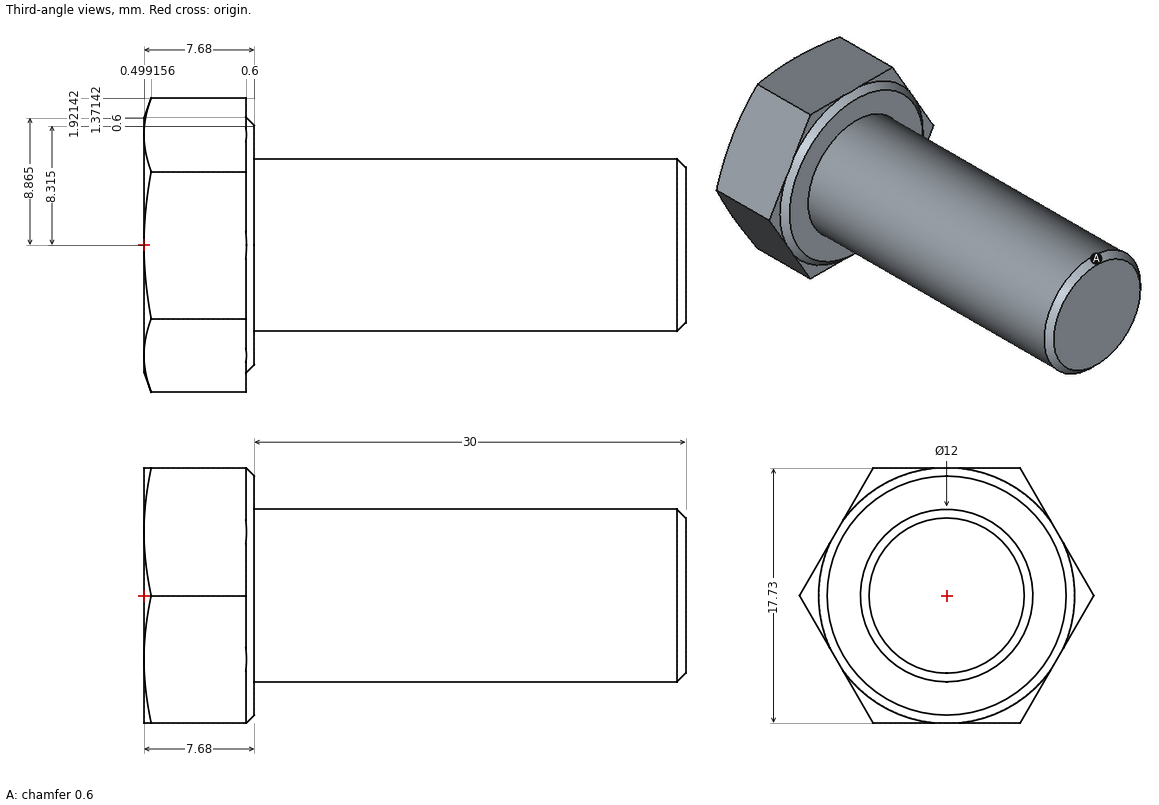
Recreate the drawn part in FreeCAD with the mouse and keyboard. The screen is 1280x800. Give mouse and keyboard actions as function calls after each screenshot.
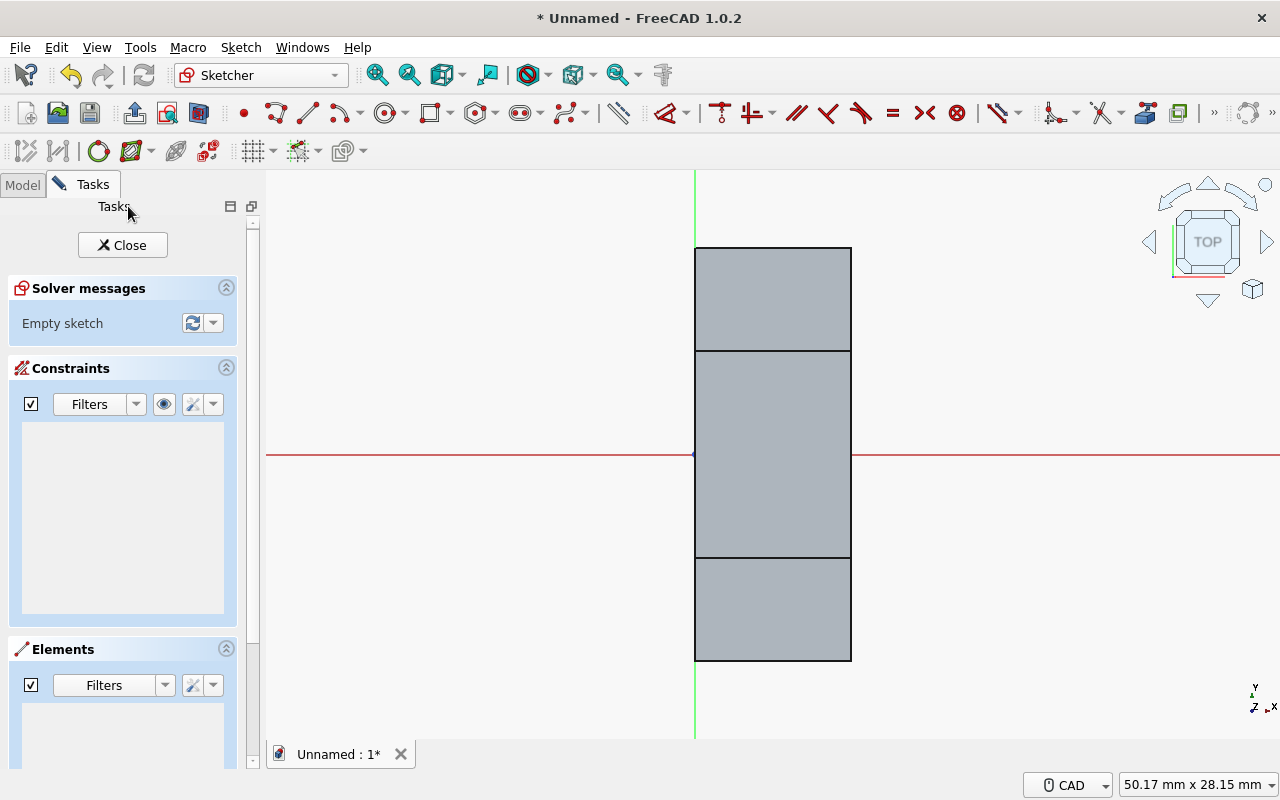
key(q)
key(s)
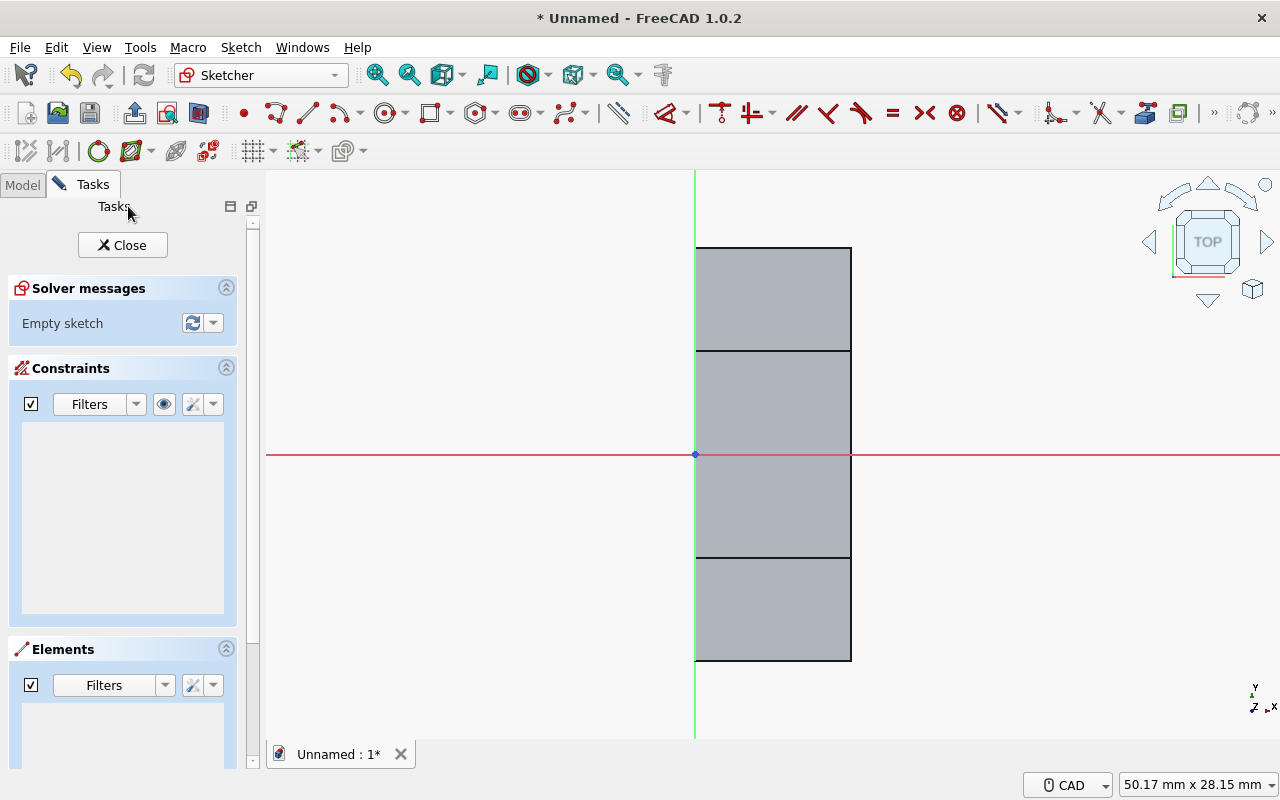
scroll(862, 244, up, 11)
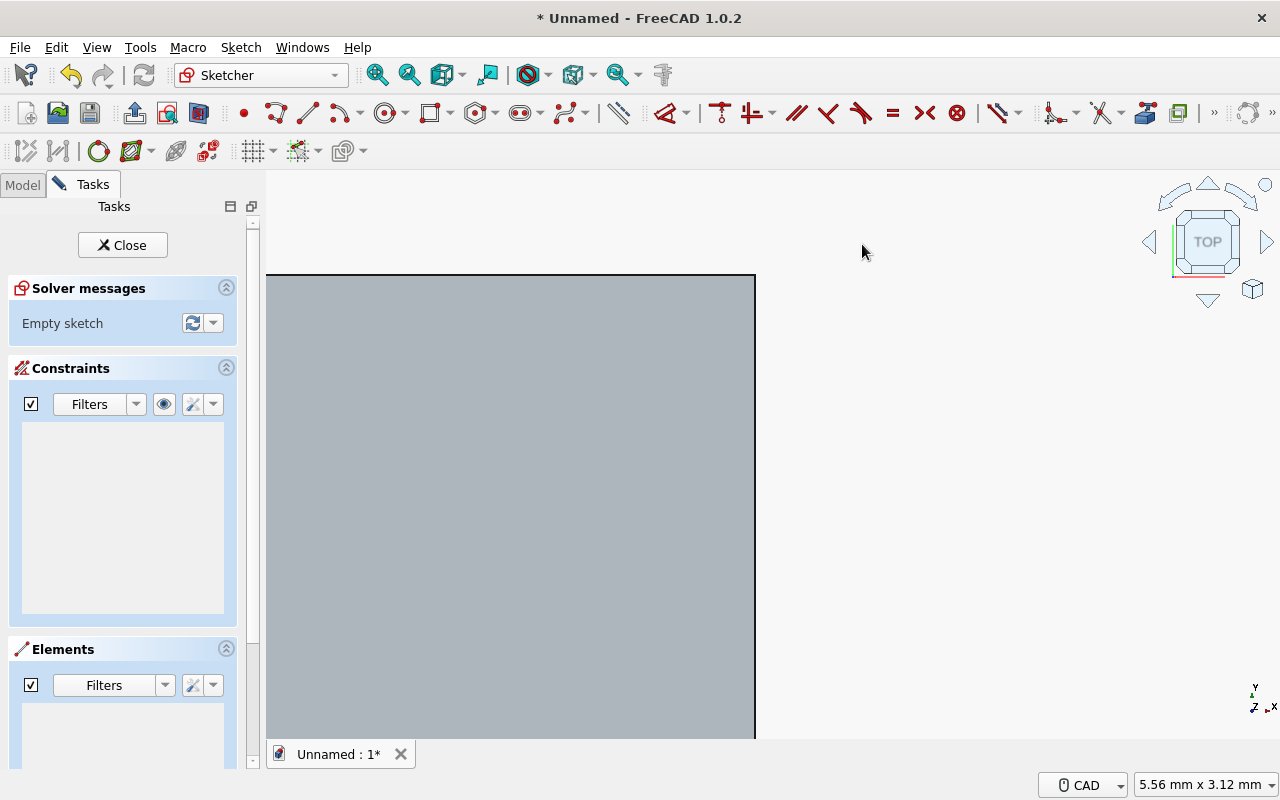
click(276, 114)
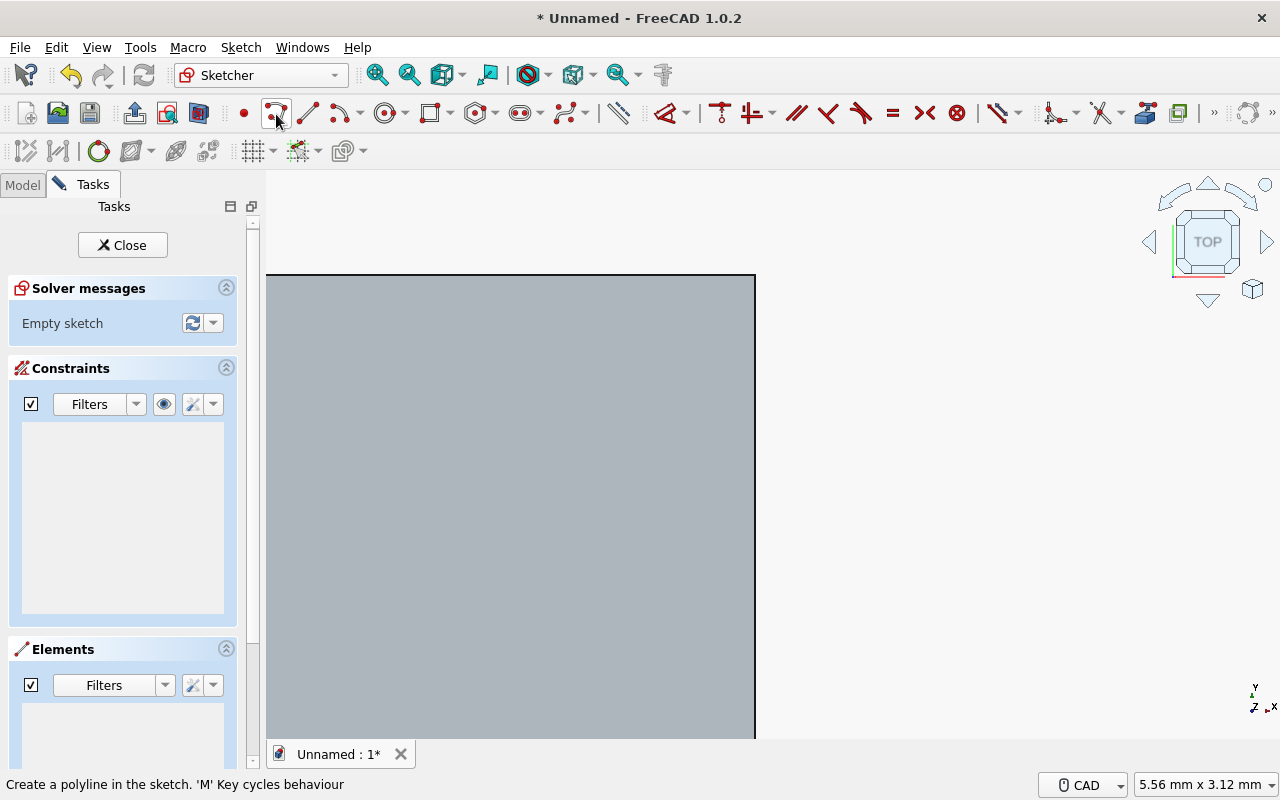
click(755, 626)
click(755, 275)
click(645, 275)
click(645, 516)
click(755, 627)
key(Escape)
key(Escape)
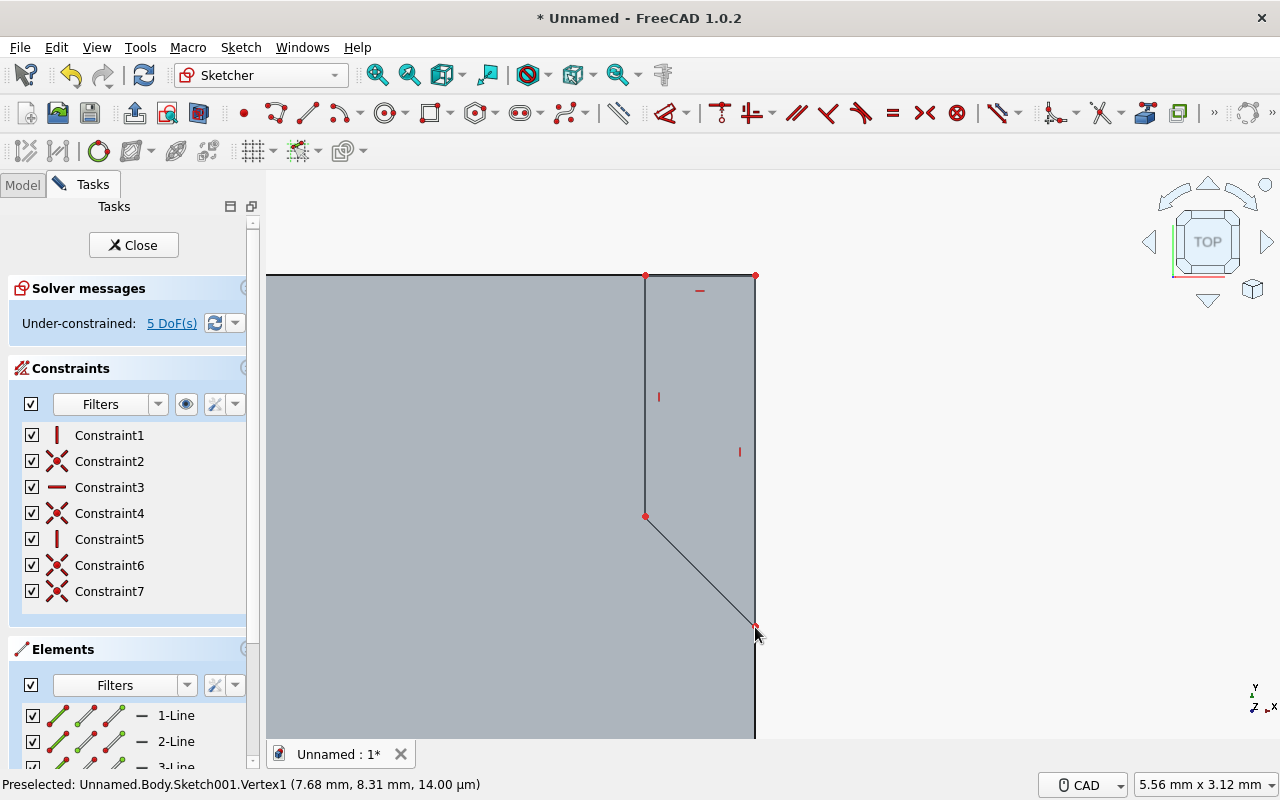
click(666, 114)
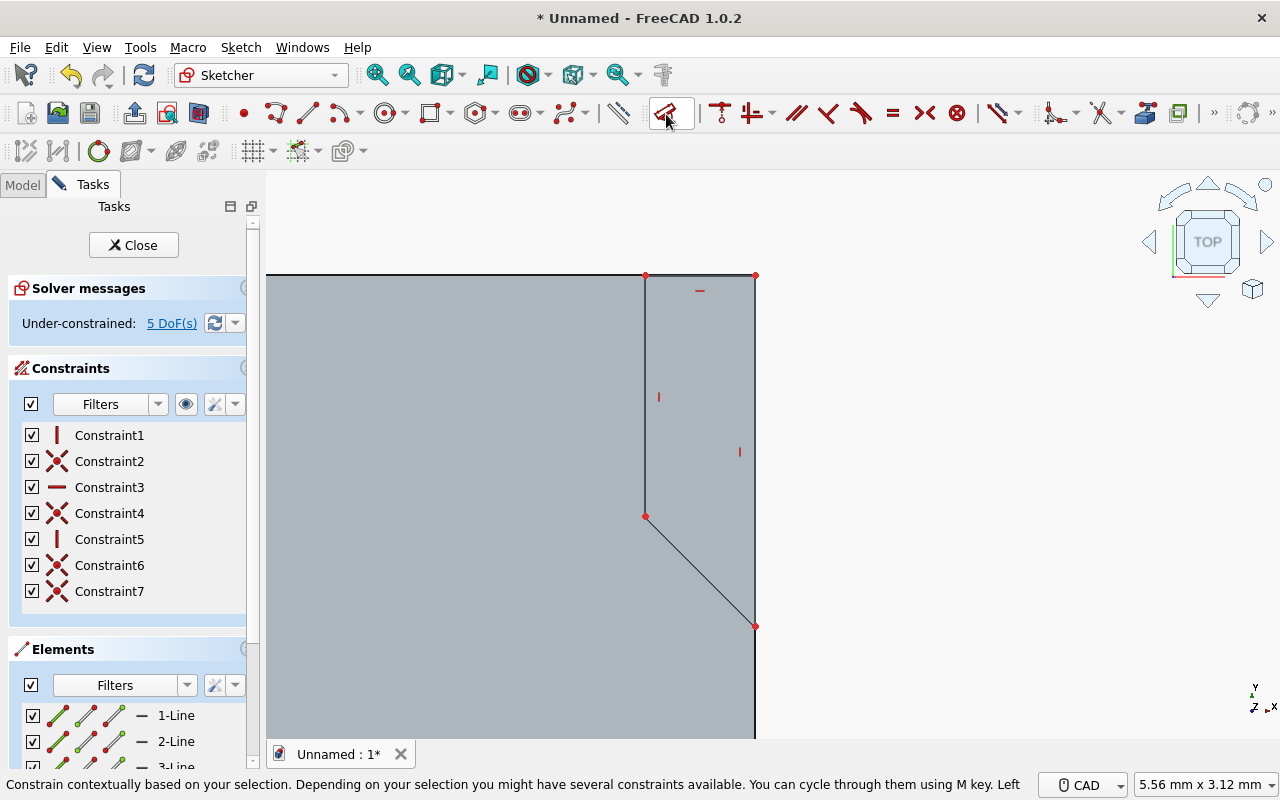
click(722, 276)
click(700, 242)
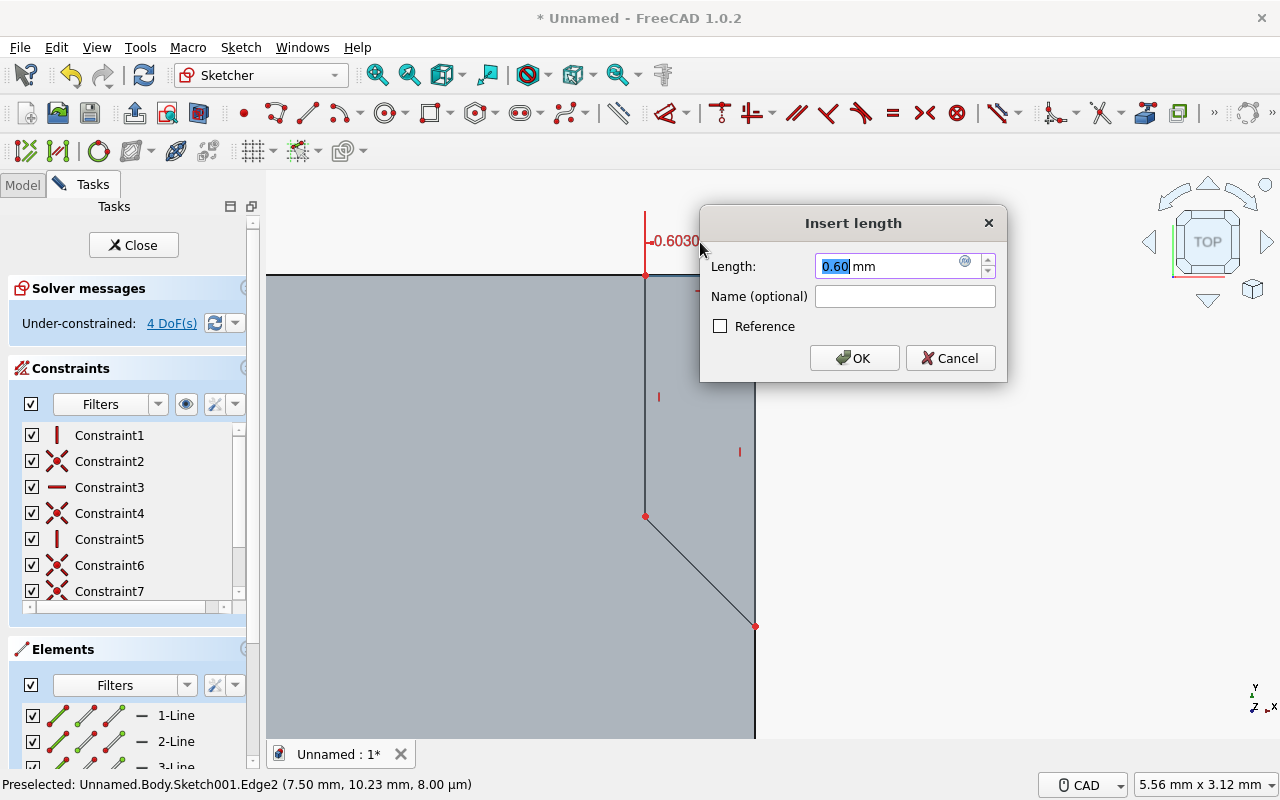
text(0.6)
key(Return)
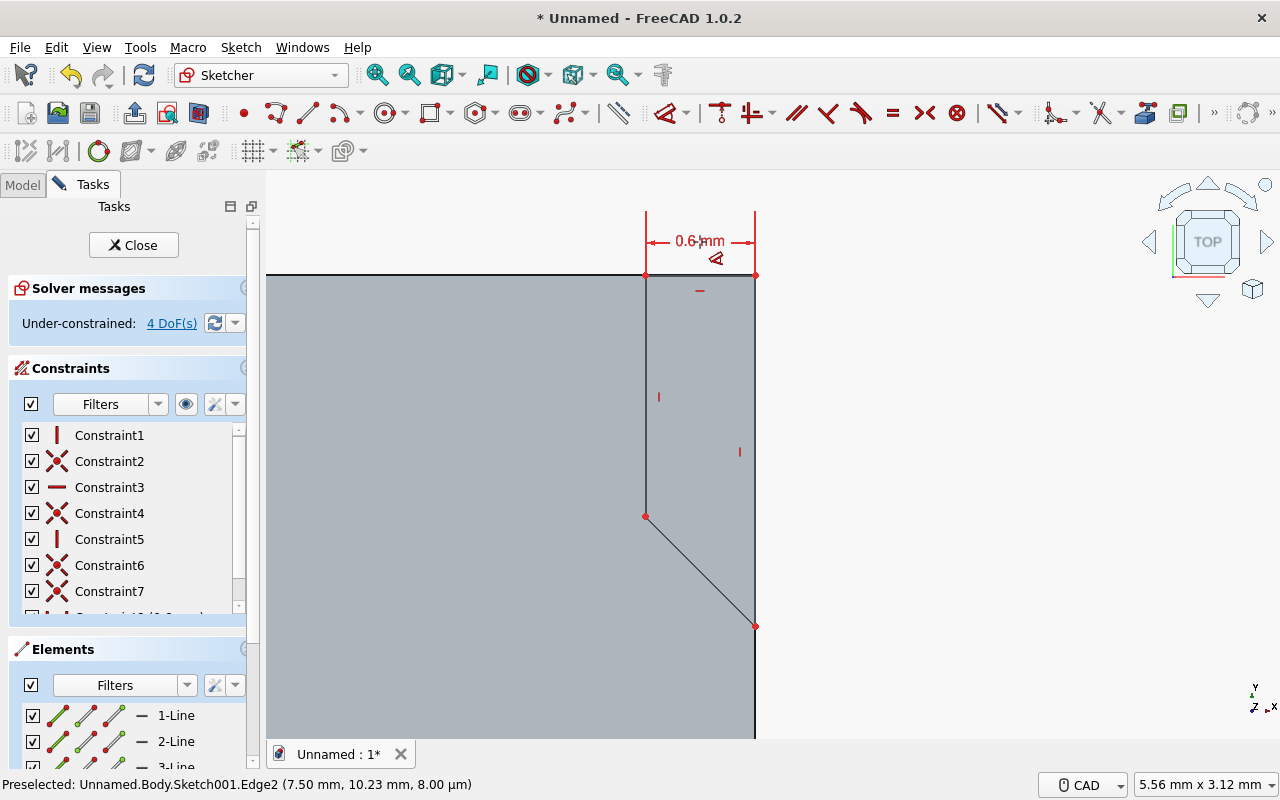
click(678, 550)
click(789, 572)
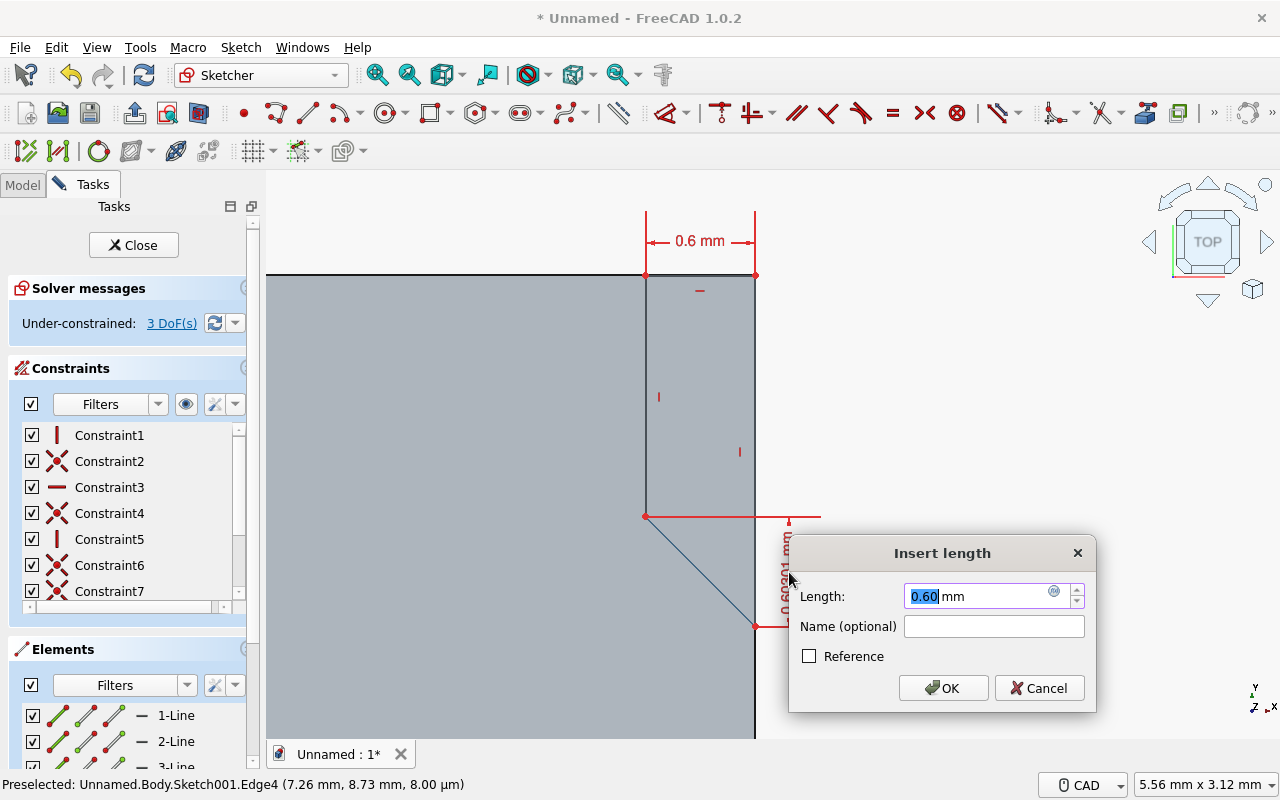
text(0.6)
key(Return)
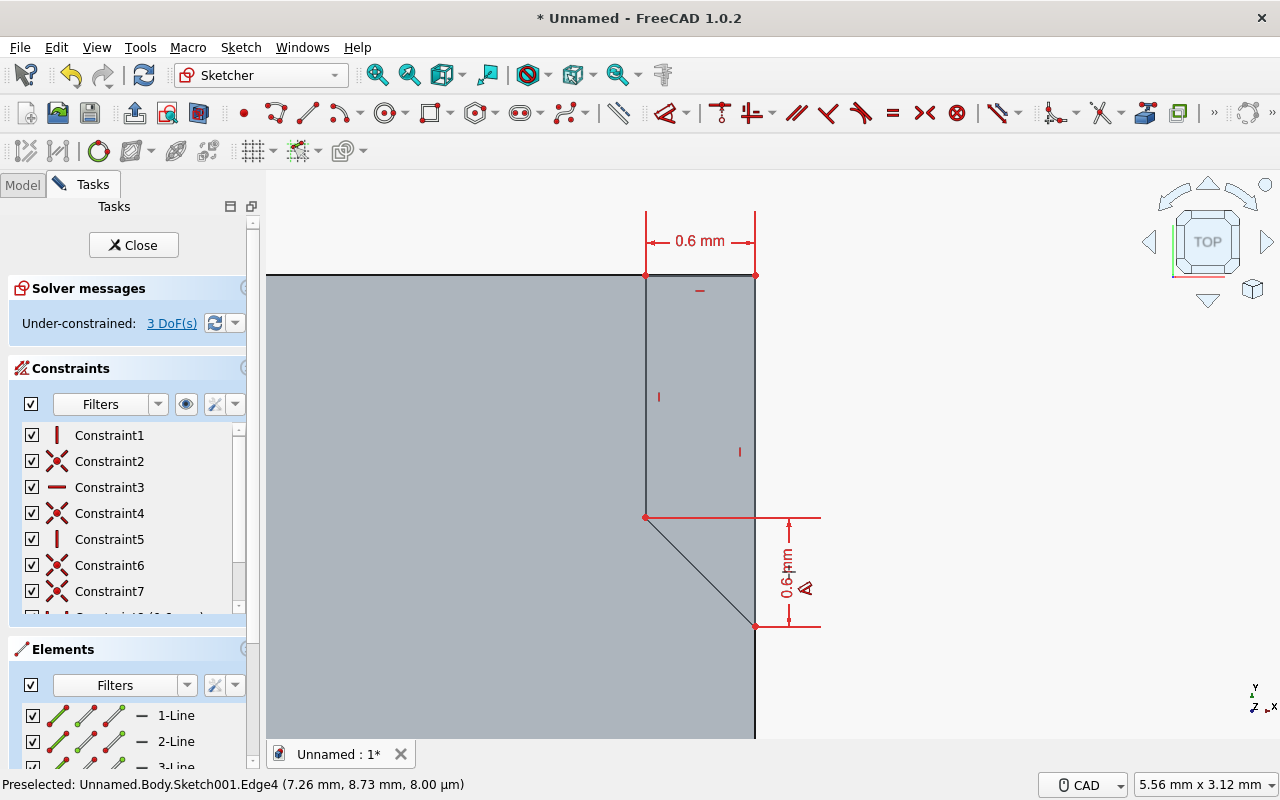
click(755, 627)
click(525, 593)